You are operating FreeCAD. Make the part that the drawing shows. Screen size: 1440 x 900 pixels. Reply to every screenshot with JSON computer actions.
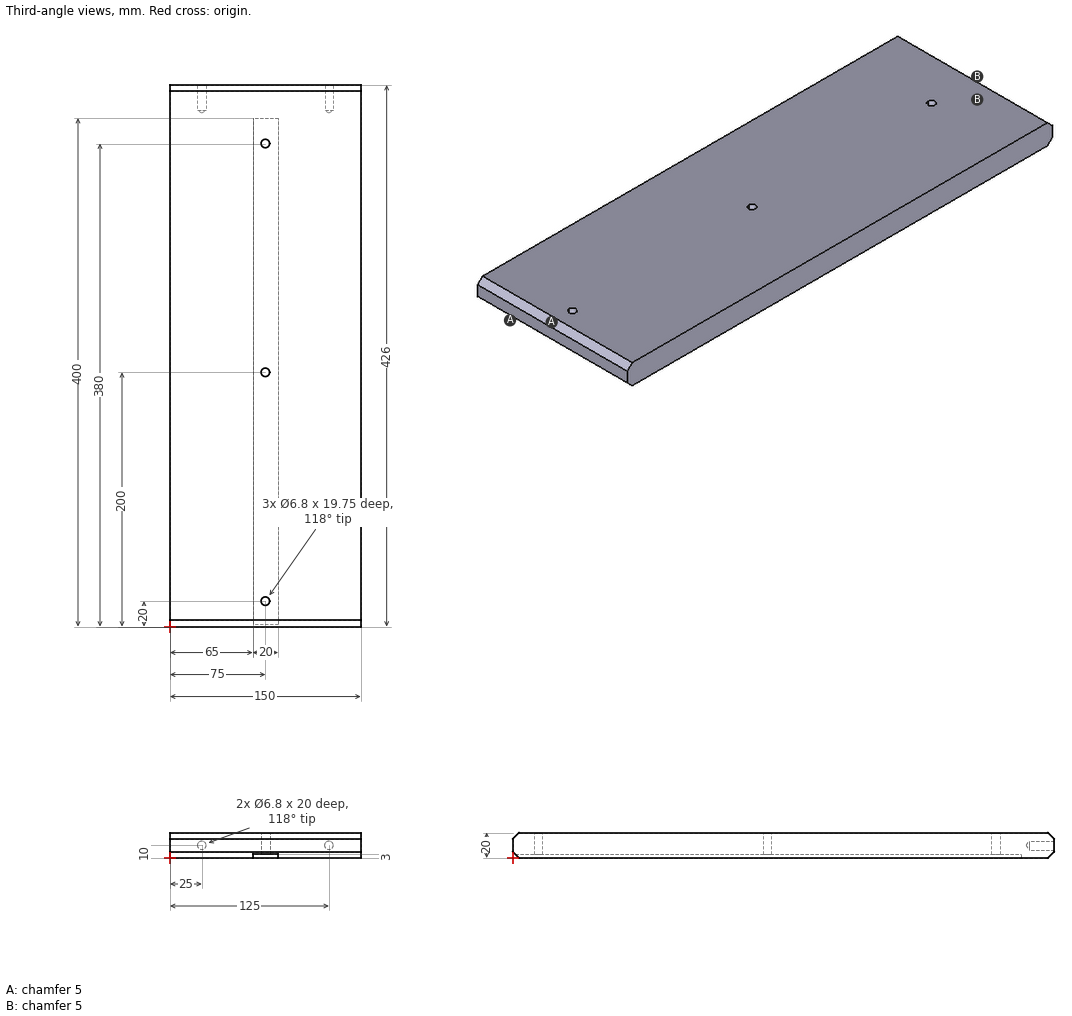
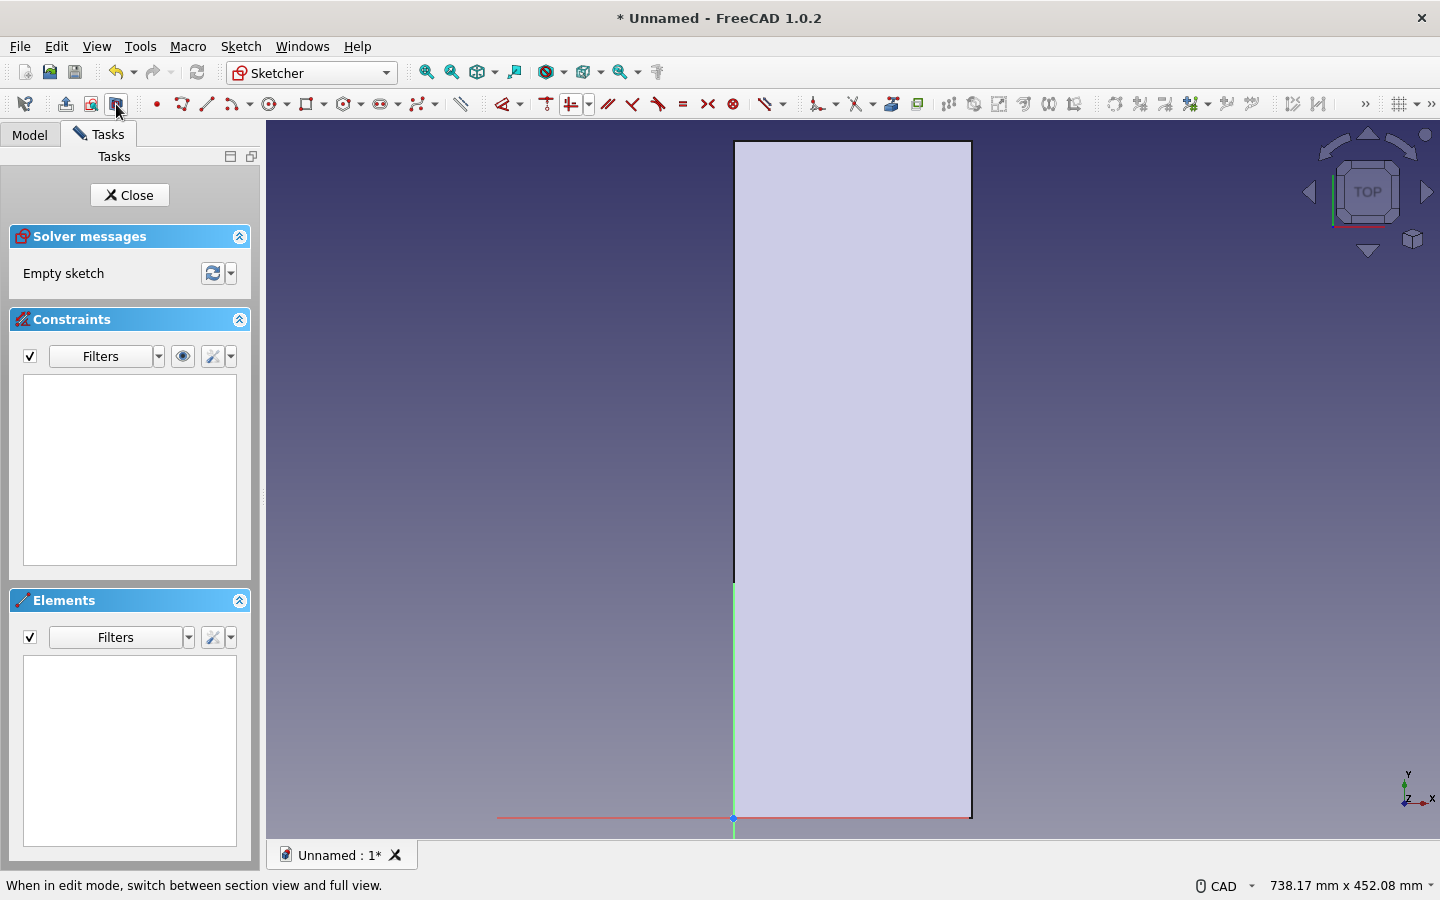
{"action": "scroll", "coordinate": [750, 437], "scroll_direction": "down", "scroll_amount": 2}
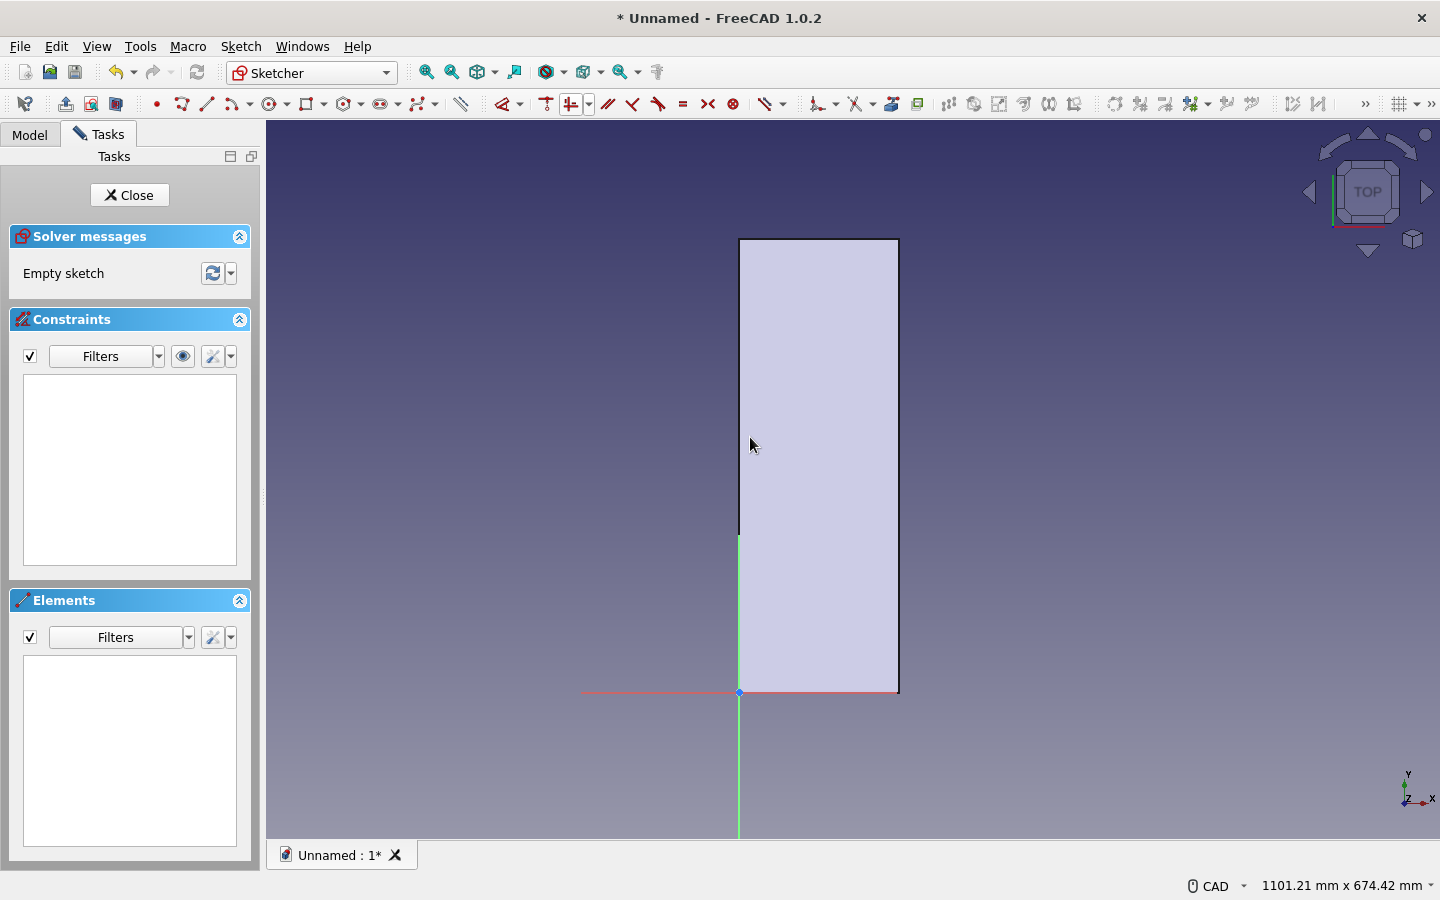
{"action": "key", "text": "g r"}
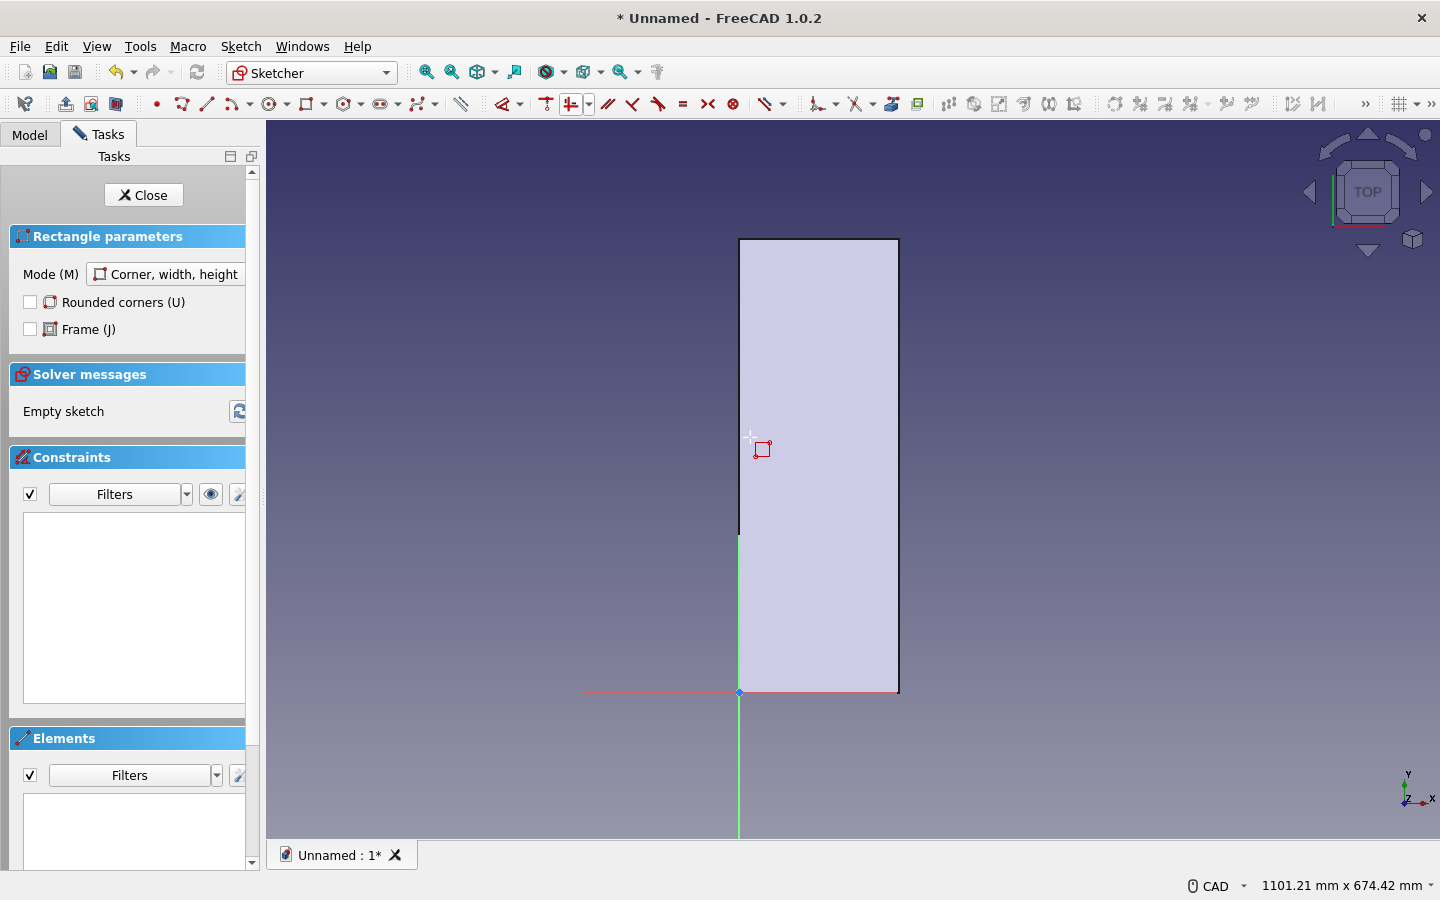
{"action": "left_click", "coordinate": [809, 266]}
{"action": "left_click", "coordinate": [830, 693]}
{"action": "key", "text": "Escape"}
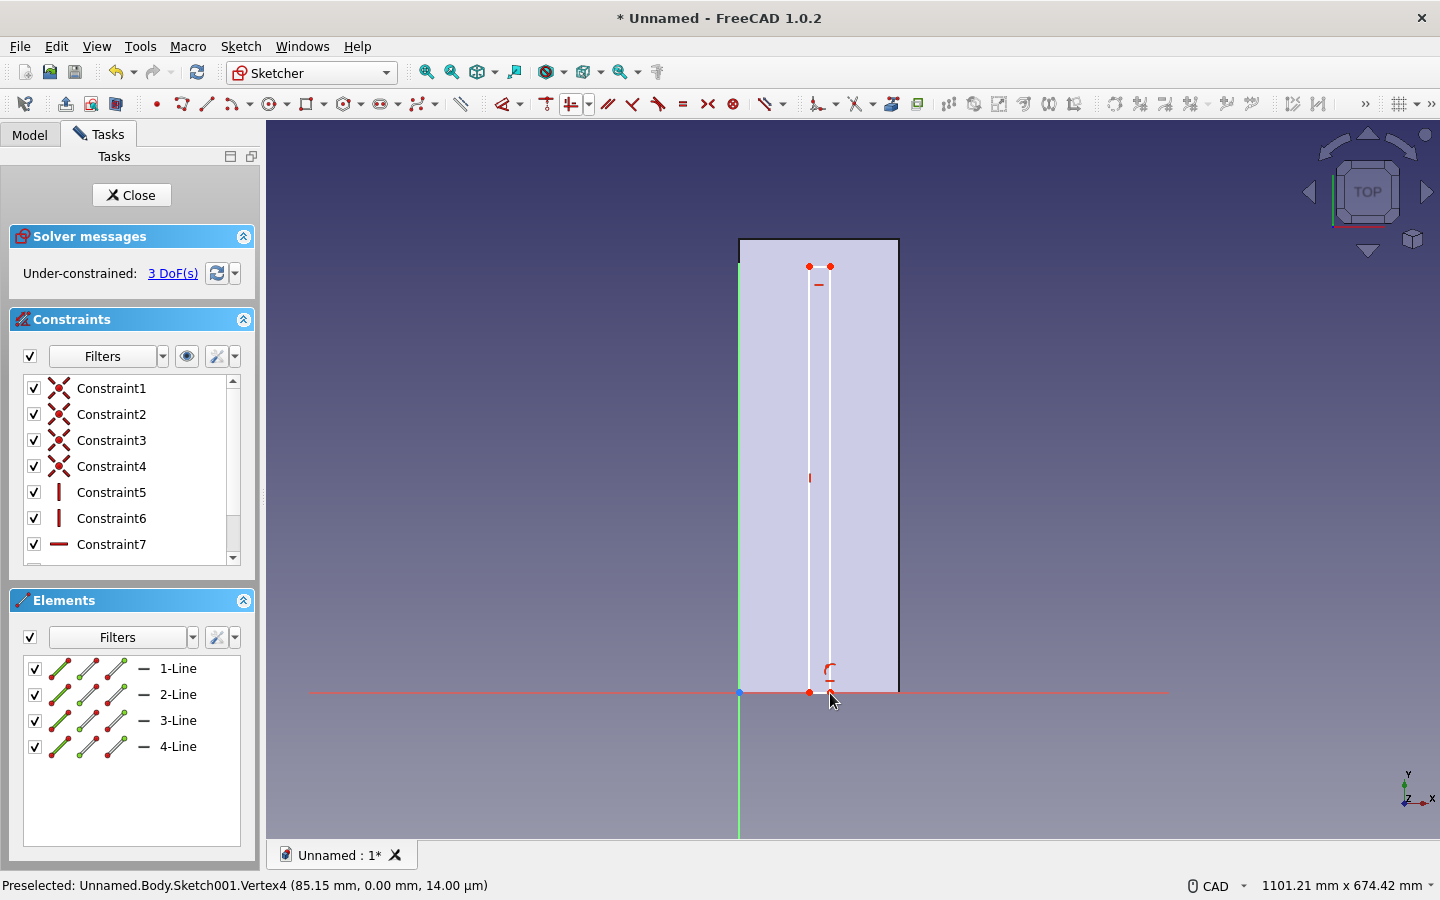
{"action": "left_click", "coordinate": [502, 104]}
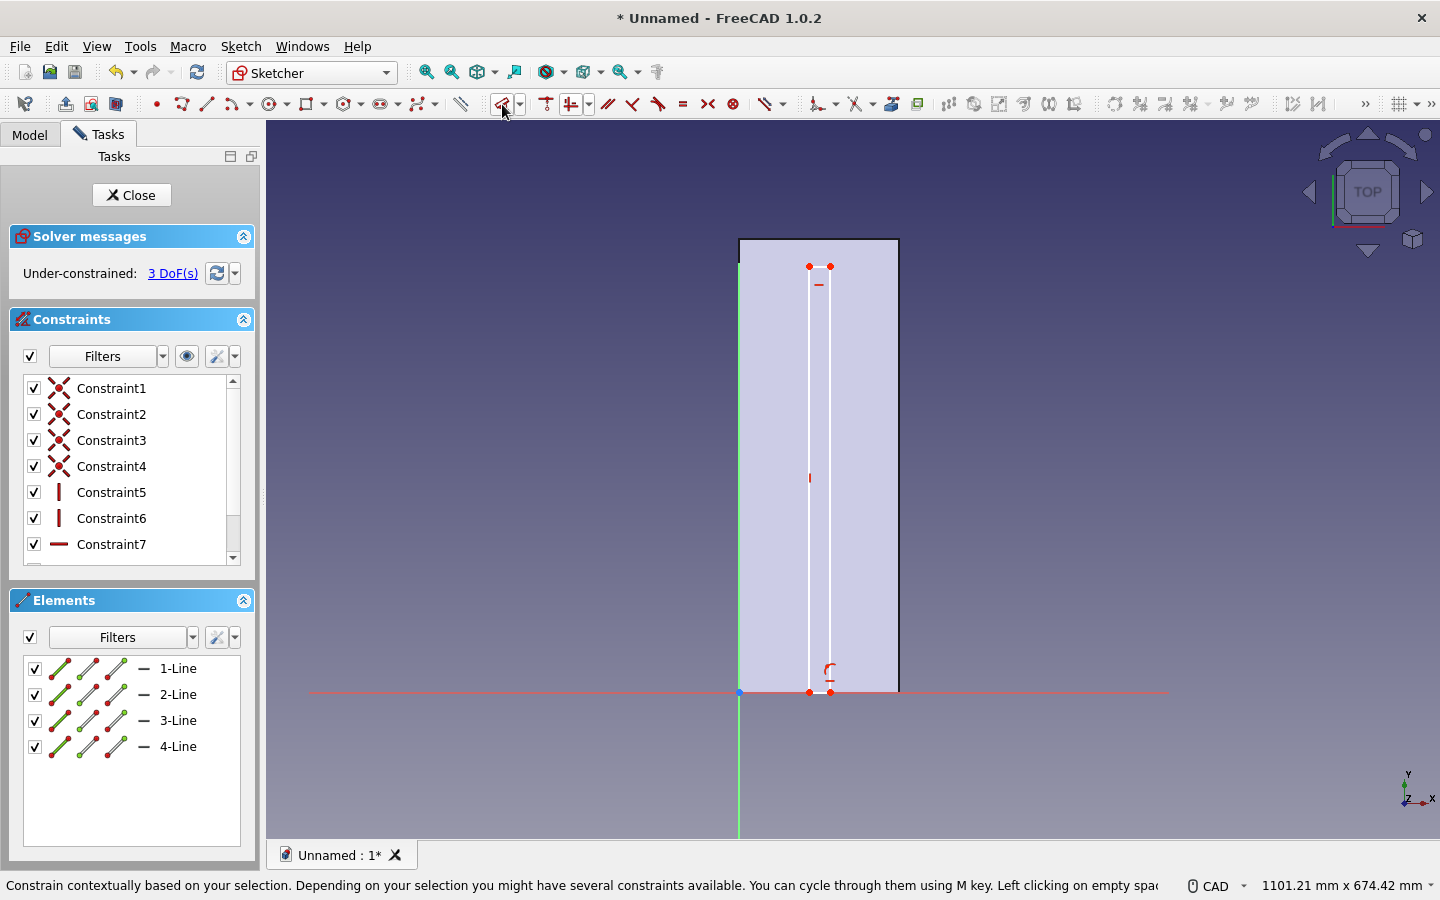
{"action": "scroll", "coordinate": [819, 693], "scroll_direction": "up", "scroll_amount": 4}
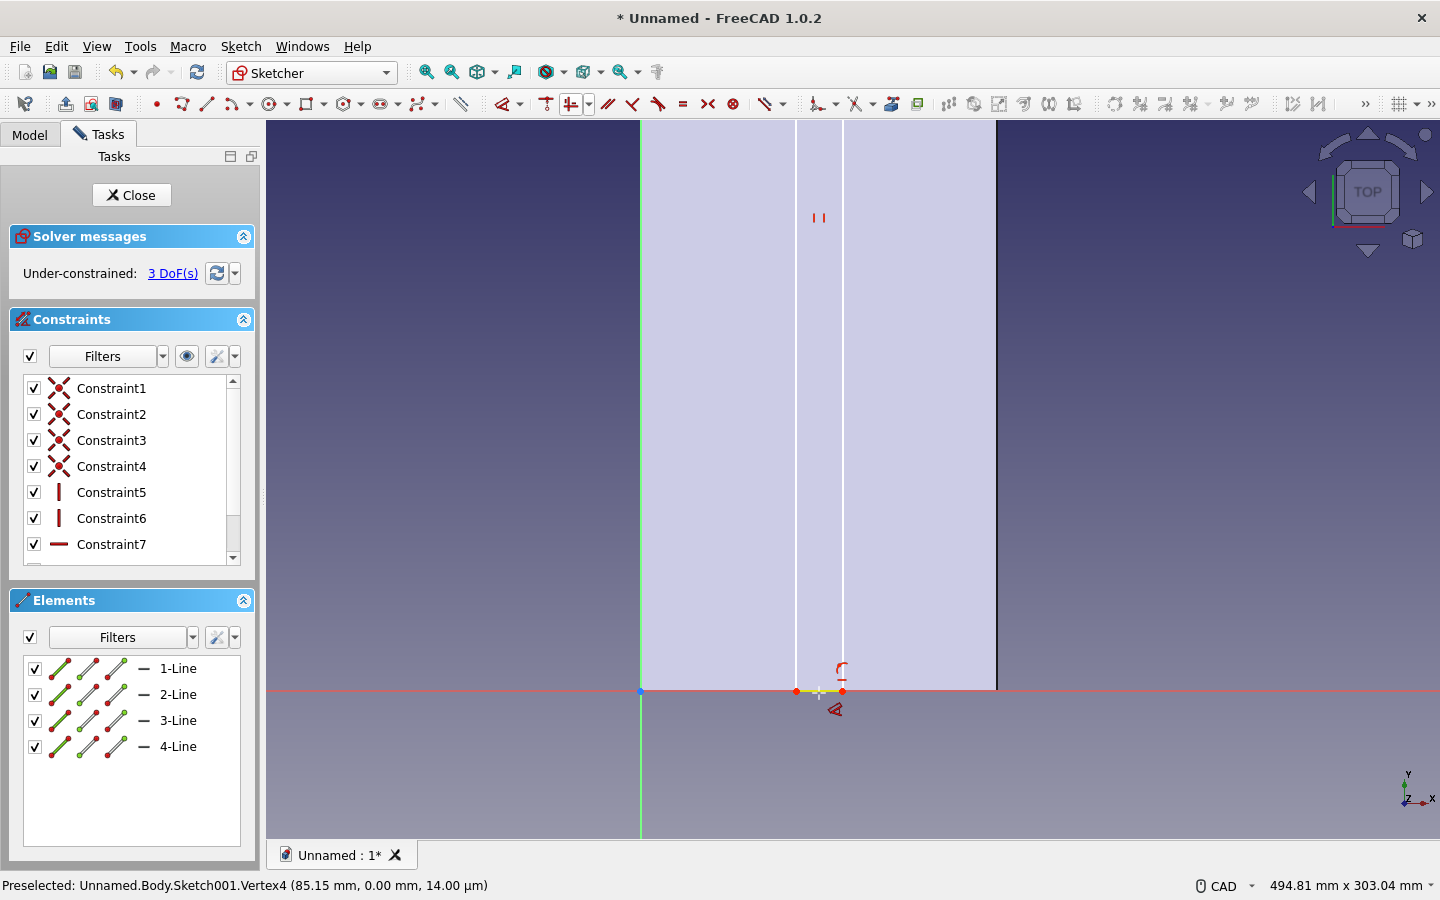
{"action": "left_click", "coordinate": [820, 691]}
{"action": "left_click", "coordinate": [820, 725]}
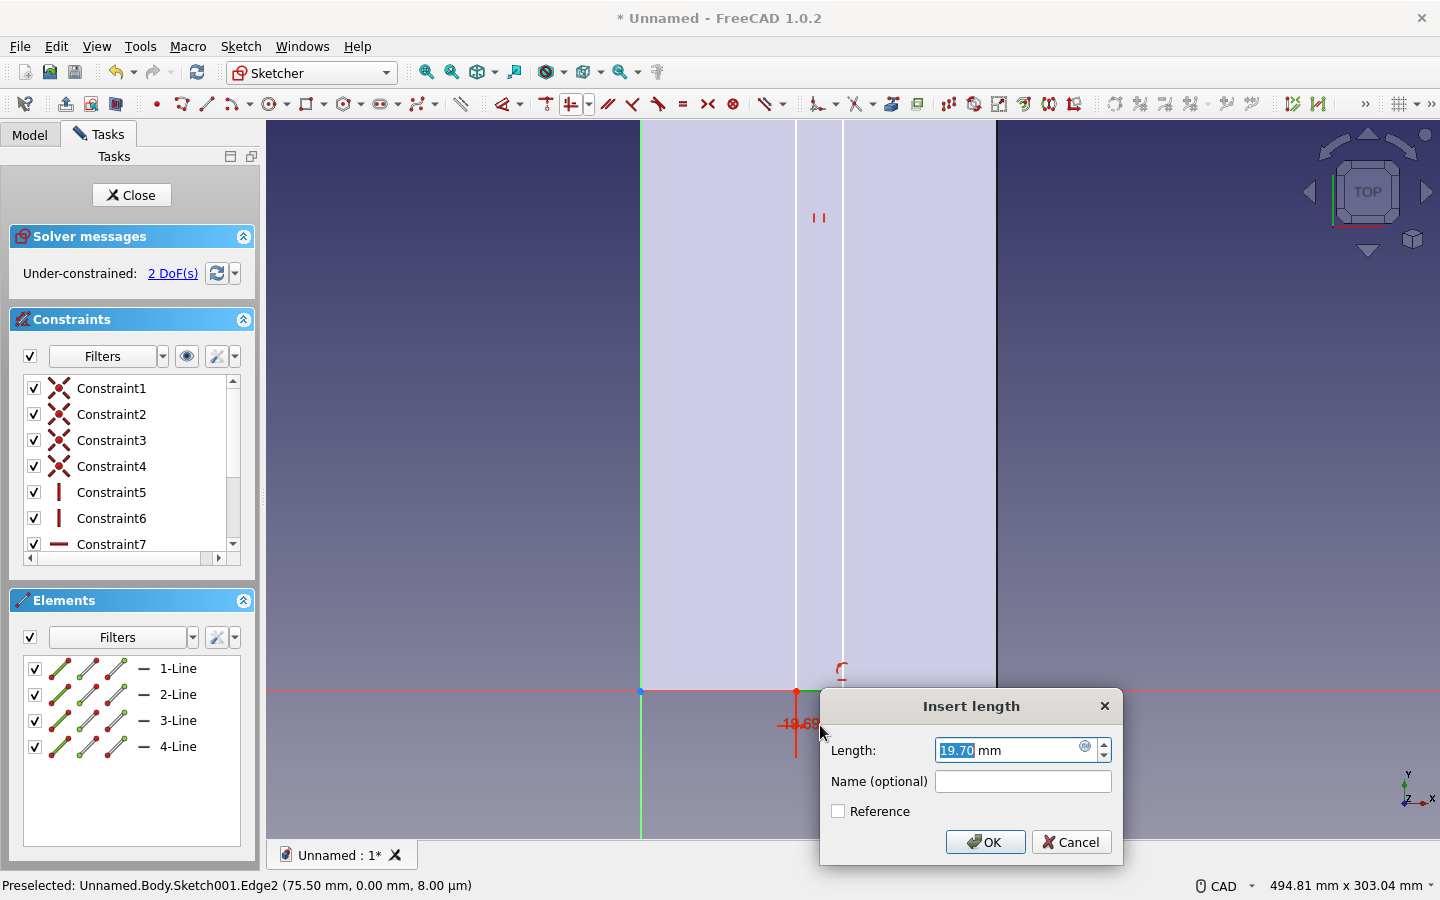
{"action": "type", "text": "20"}
{"action": "key", "text": "Return"}